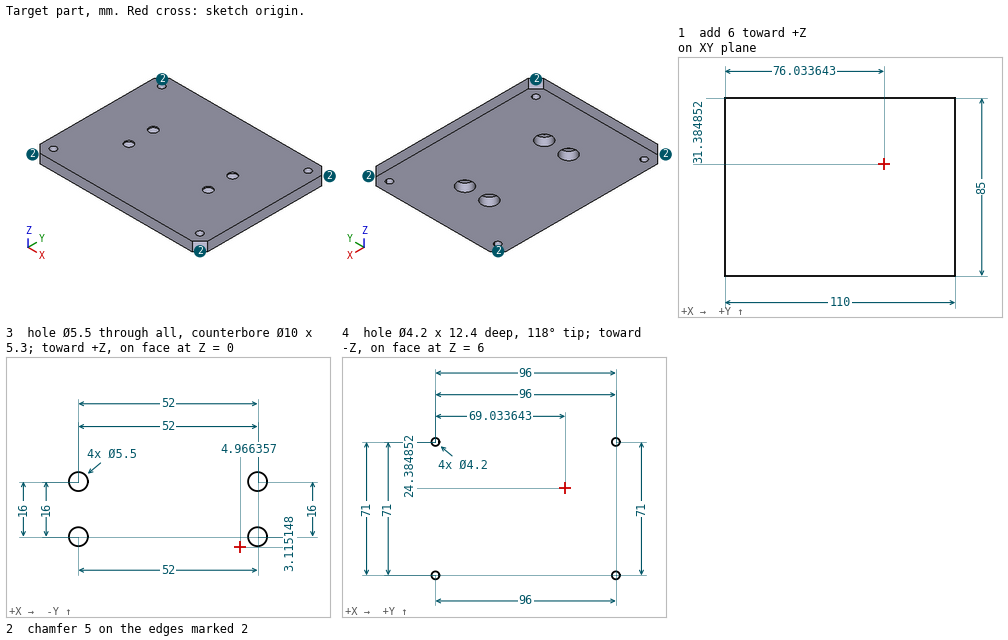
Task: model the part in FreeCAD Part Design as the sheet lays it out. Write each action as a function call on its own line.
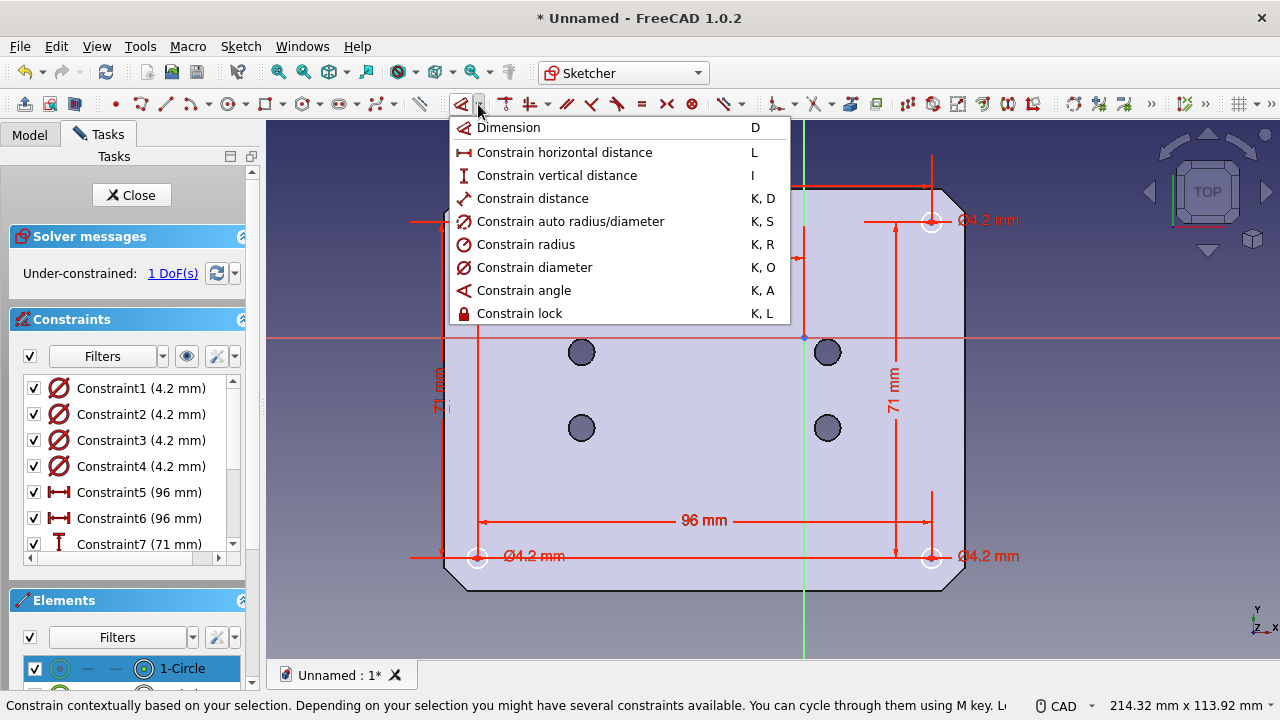
click(620, 176)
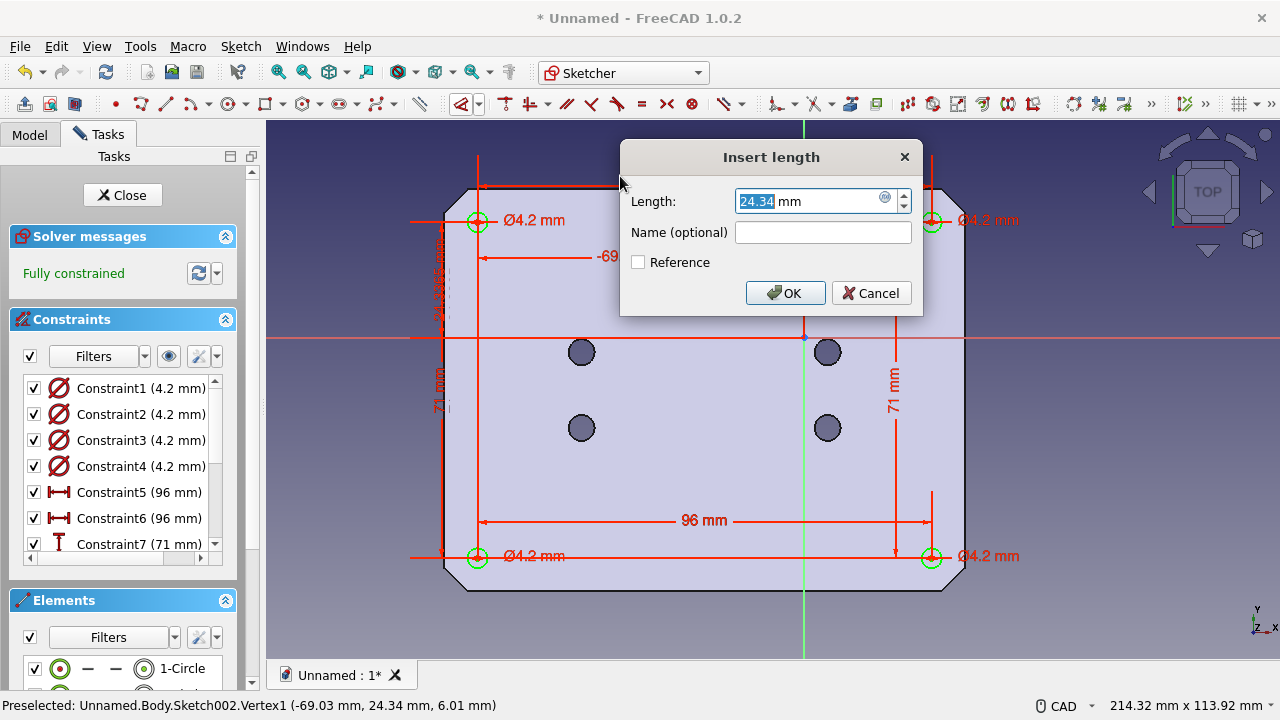
text(24.384852)
key(Return)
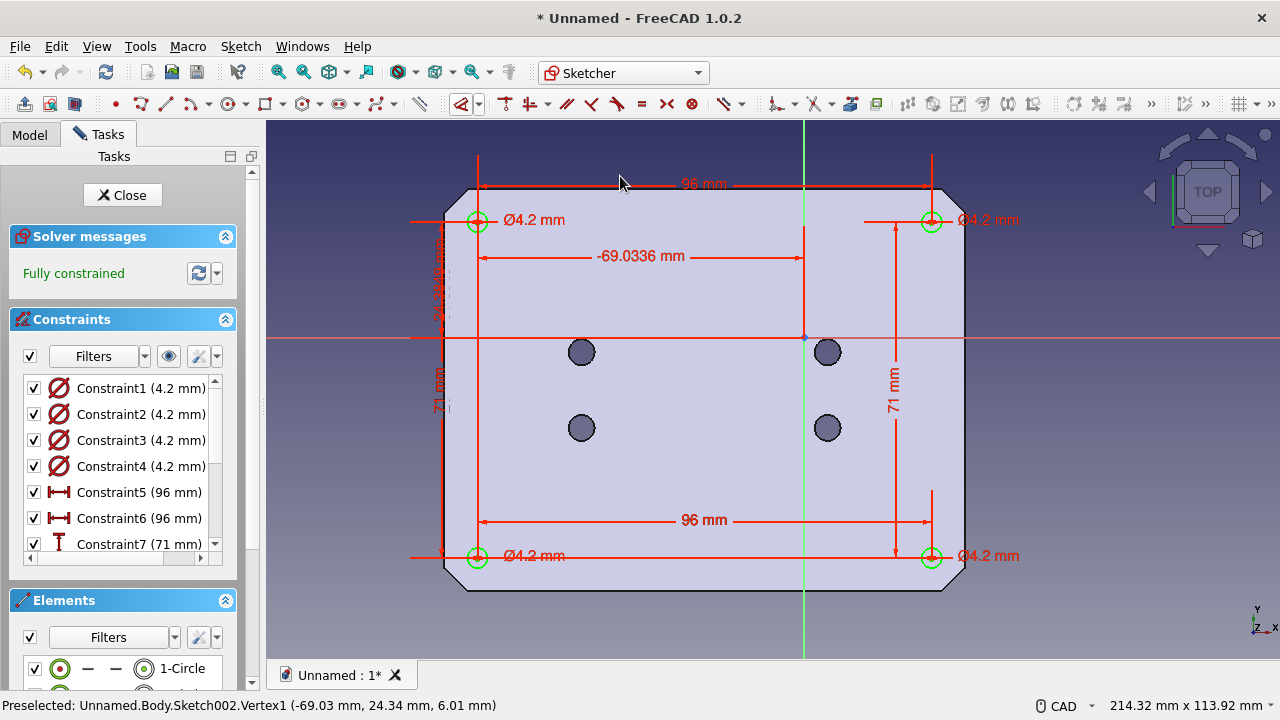
click(123, 195)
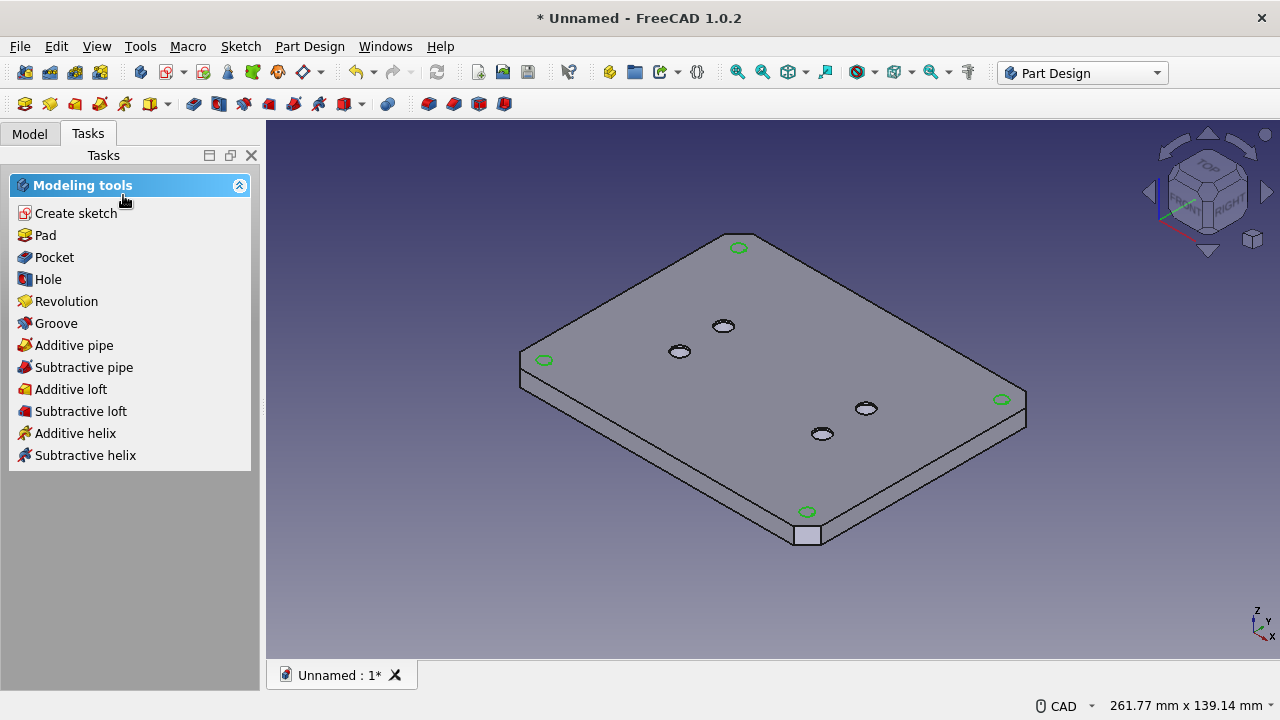
click(219, 104)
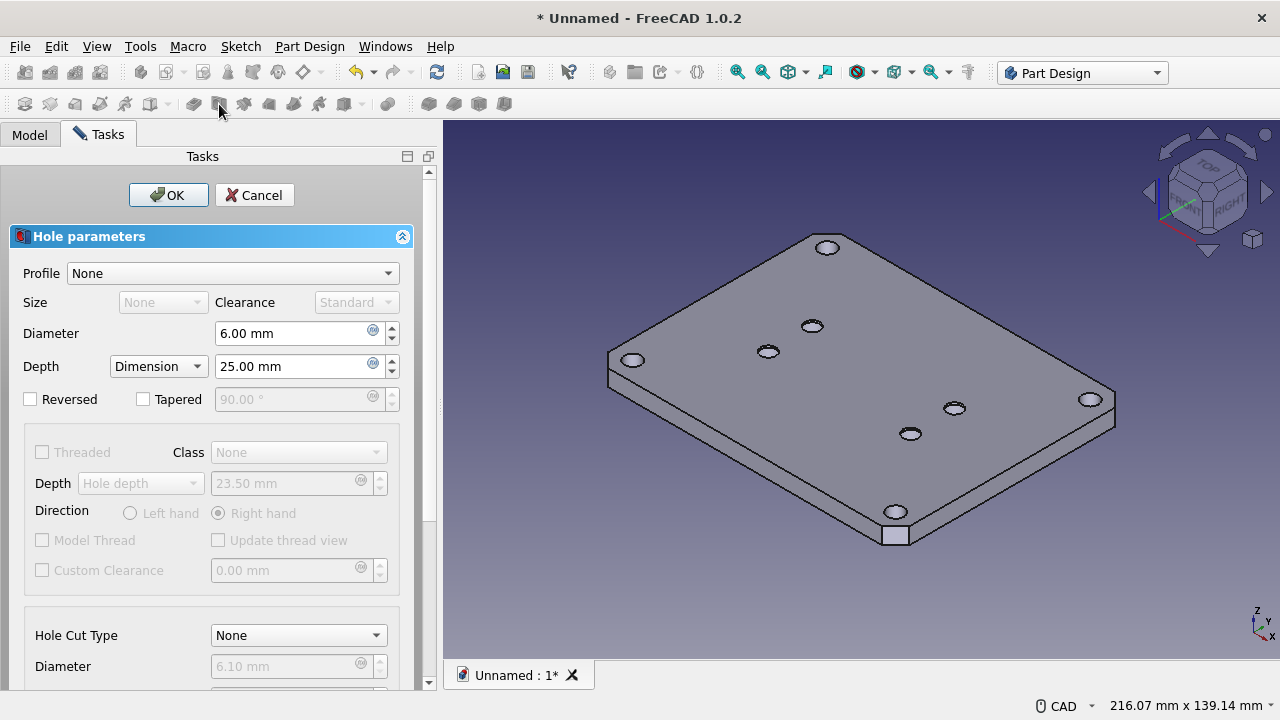
triple_click(300, 334)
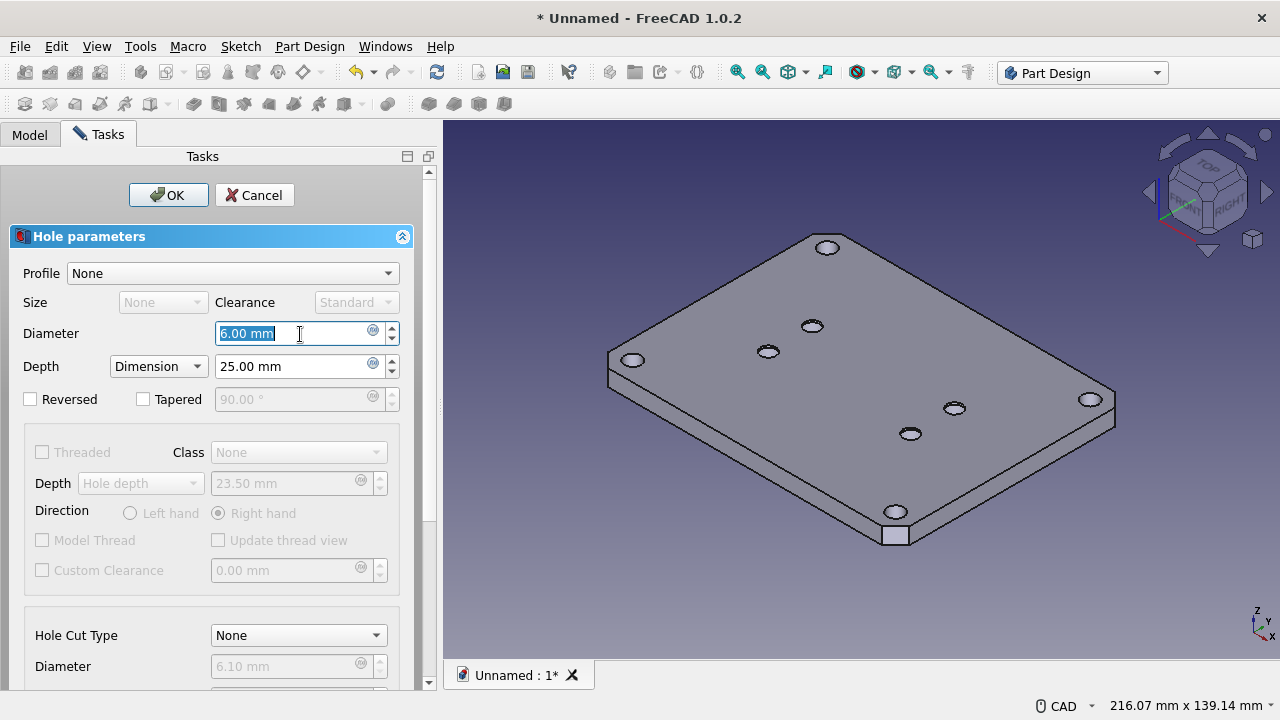
text(4.2)
key(Tab)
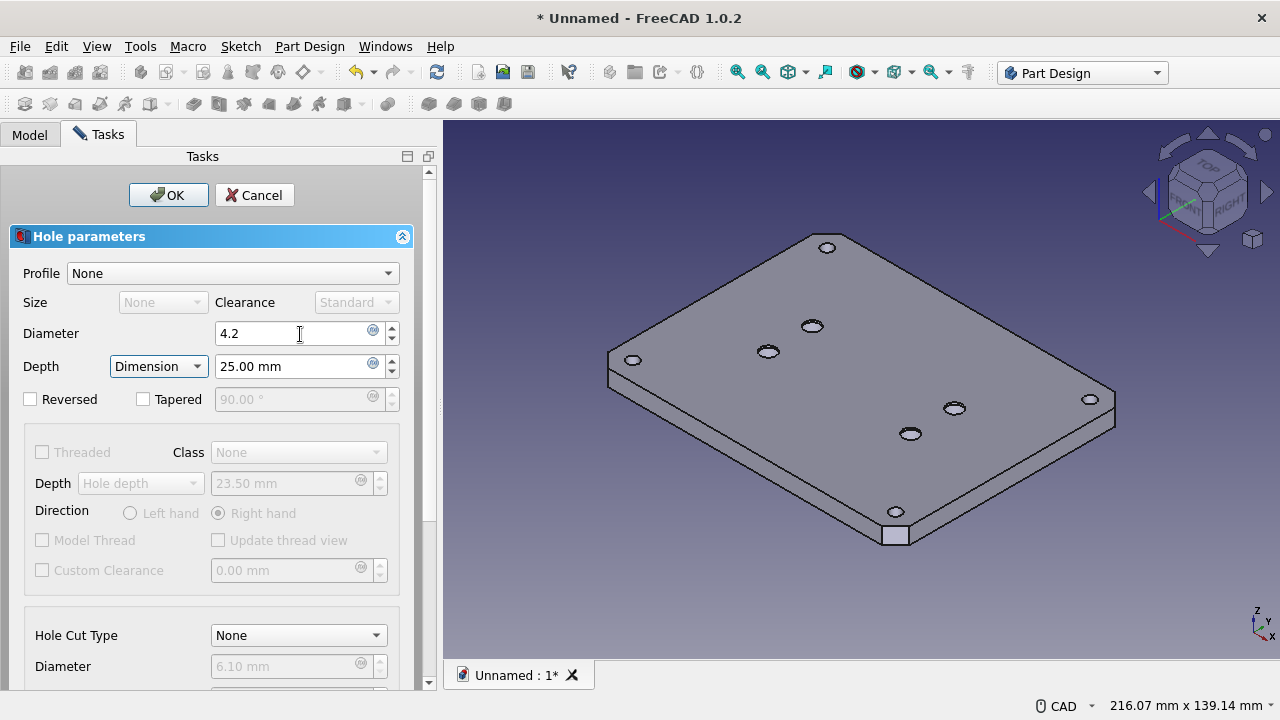
triple_click(300, 366)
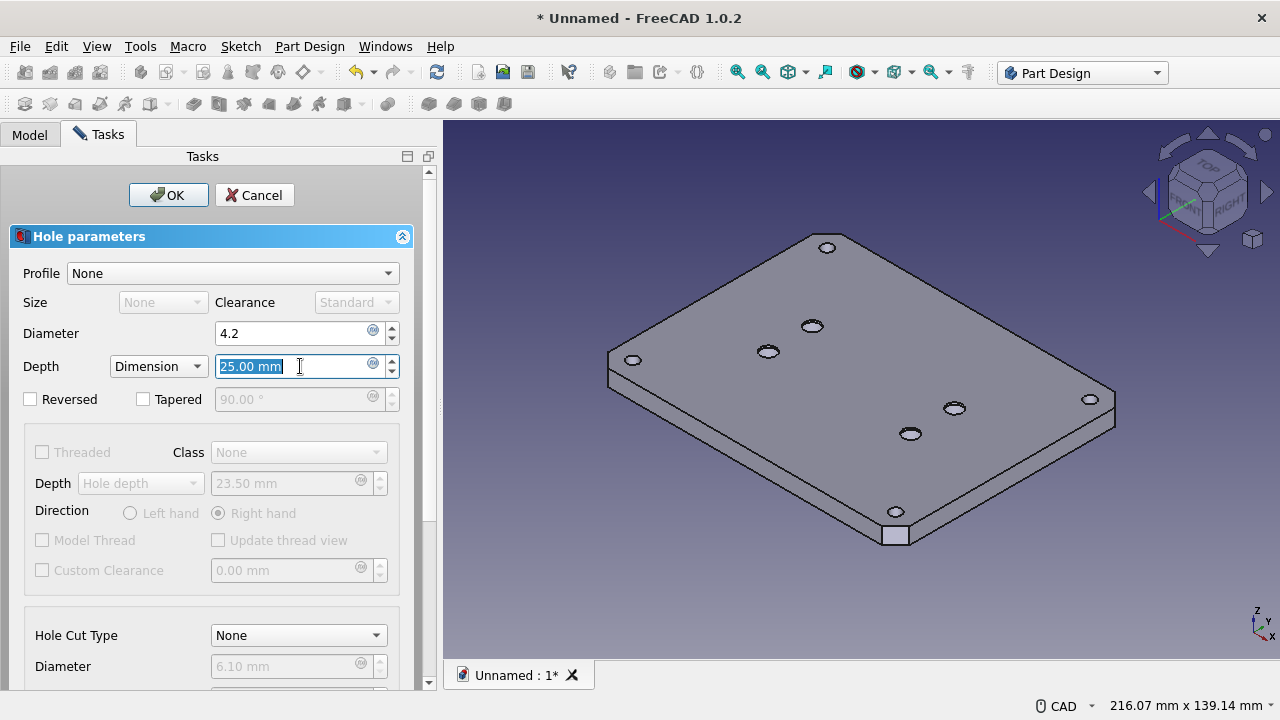
text(12.4)
key(Tab)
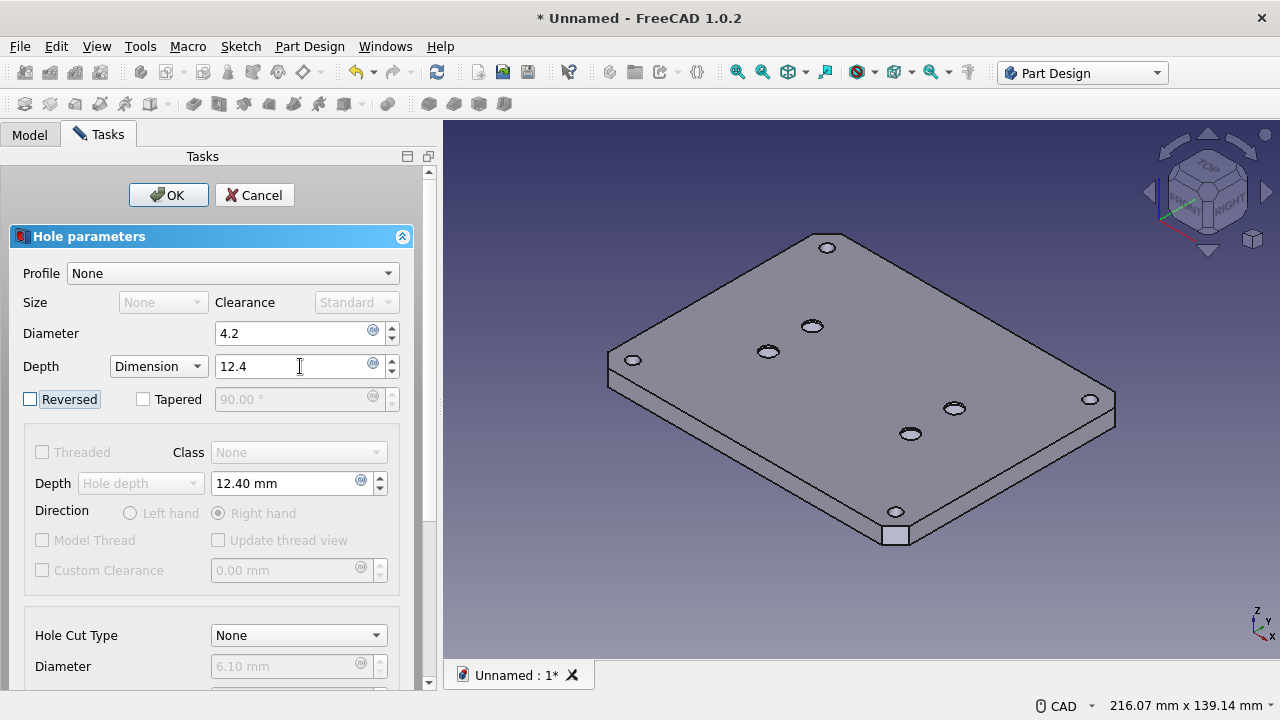
click(169, 195)